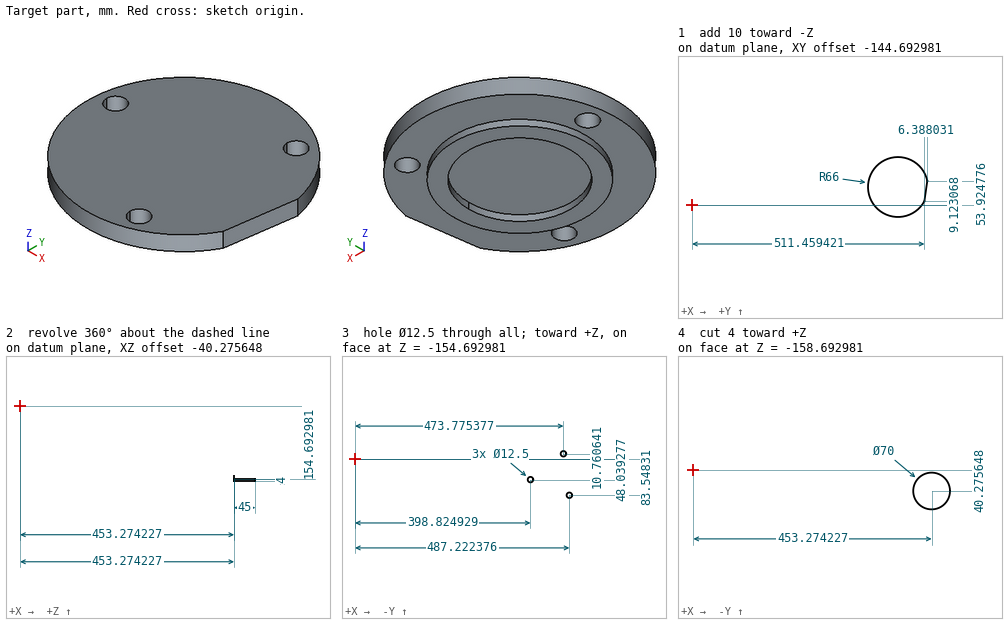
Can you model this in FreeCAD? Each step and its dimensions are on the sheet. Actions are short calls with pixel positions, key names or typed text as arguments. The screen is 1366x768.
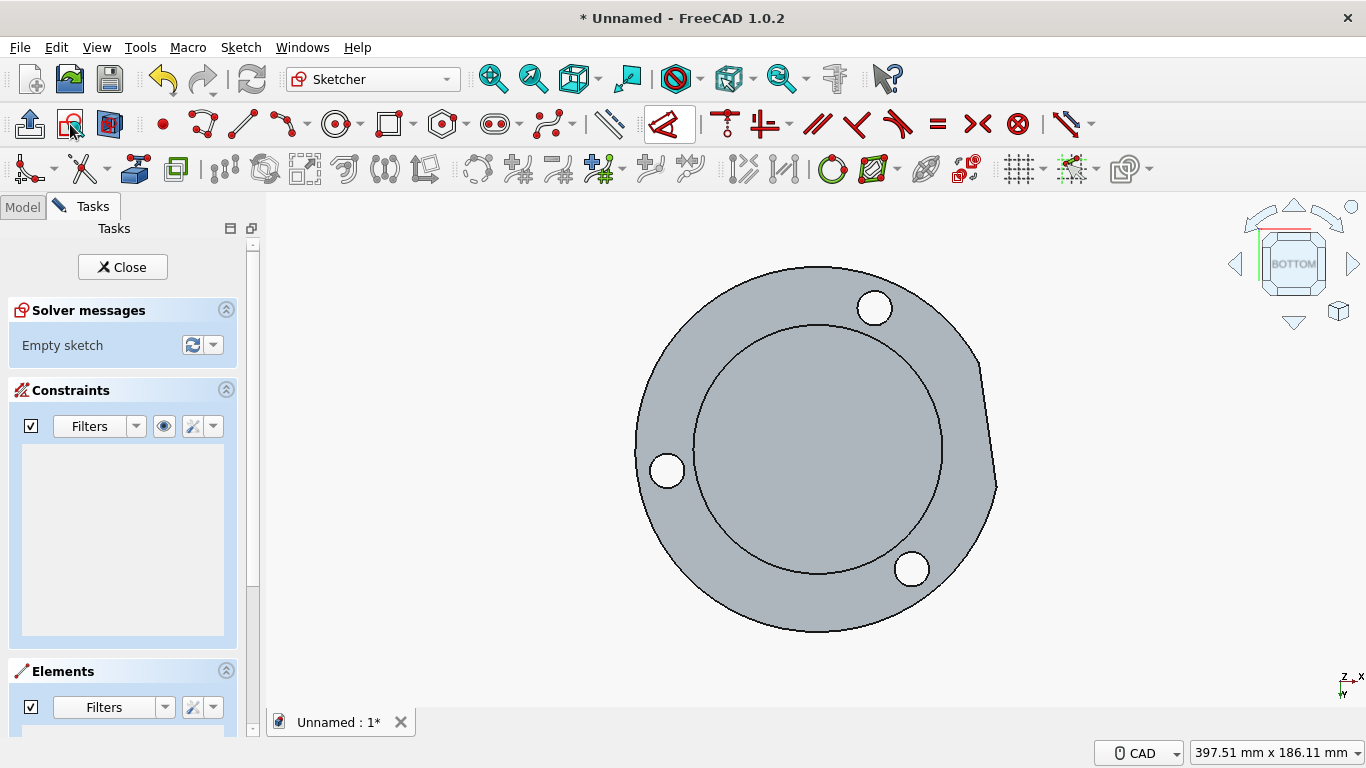
scroll(904, 449, up, 3)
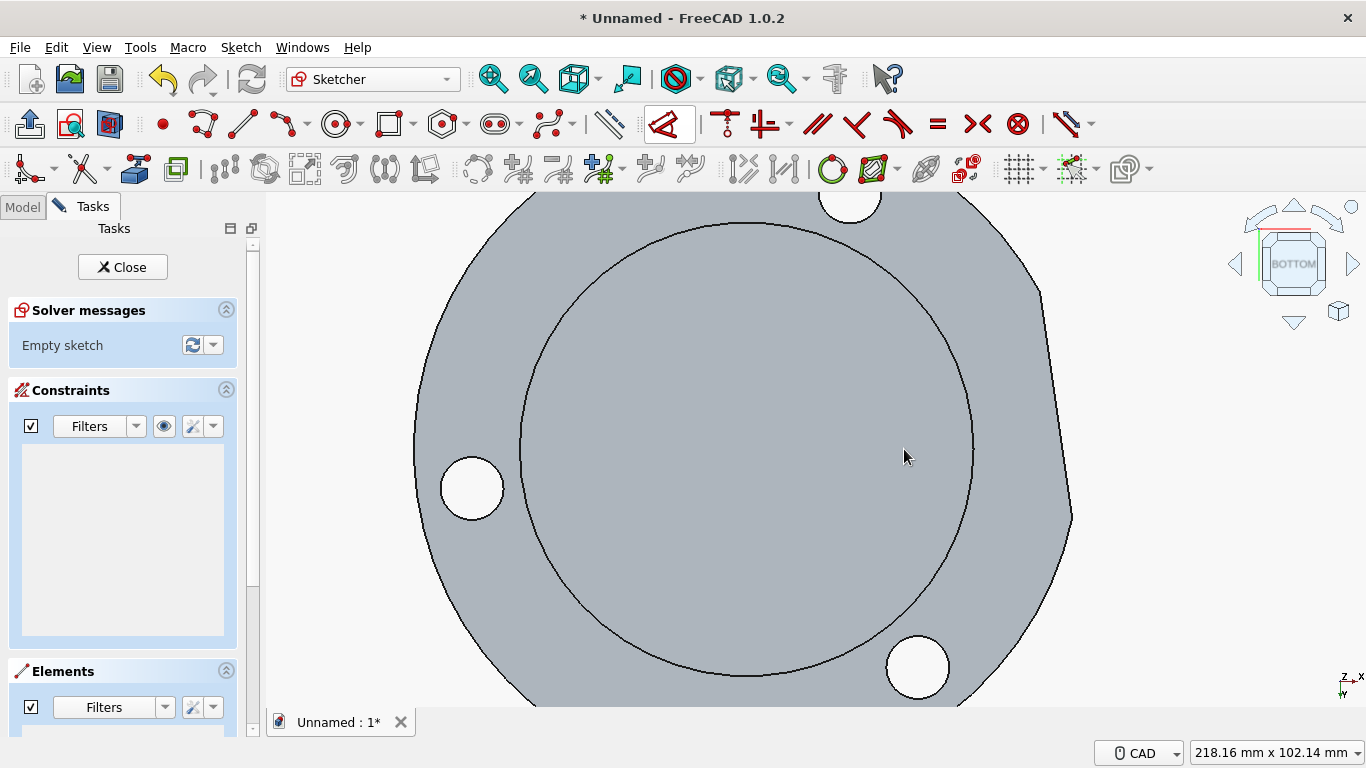
key(g)
key(c)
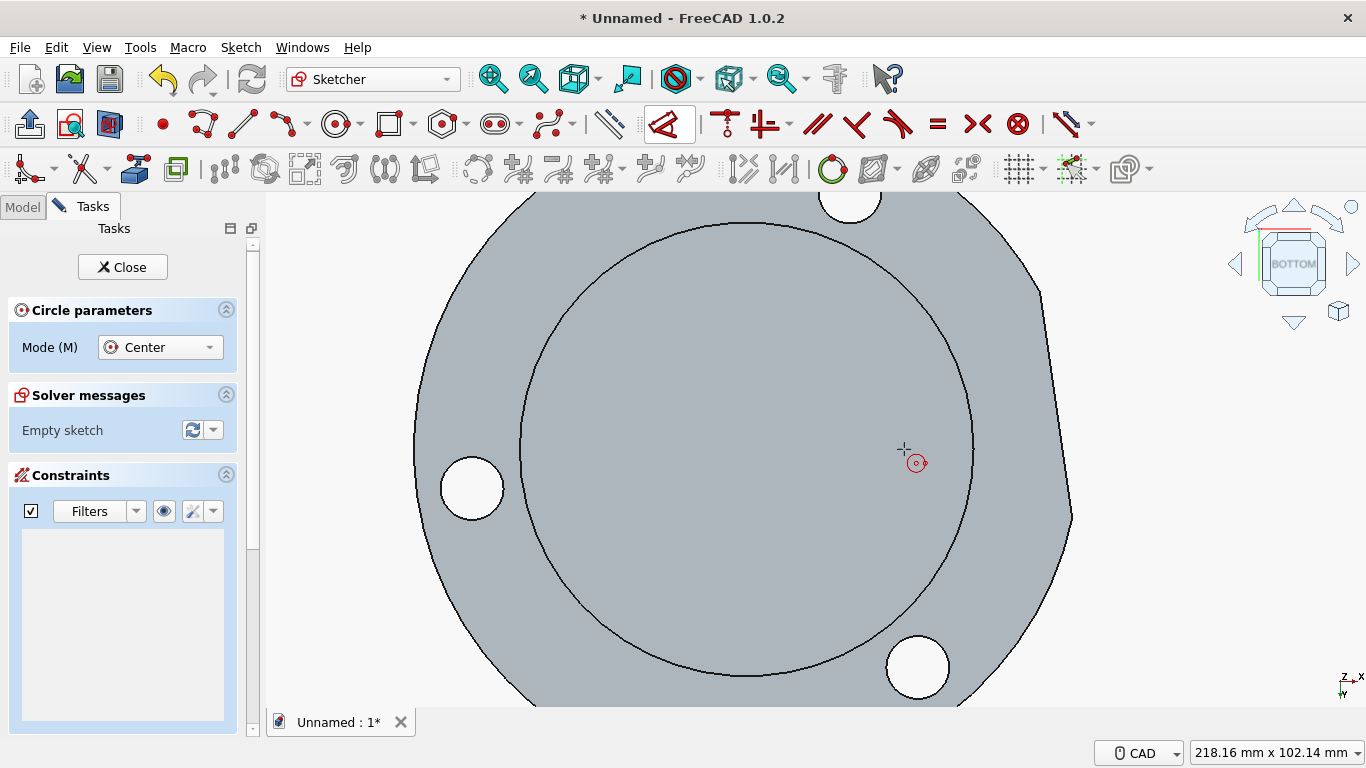
click(747, 449)
move(871, 325)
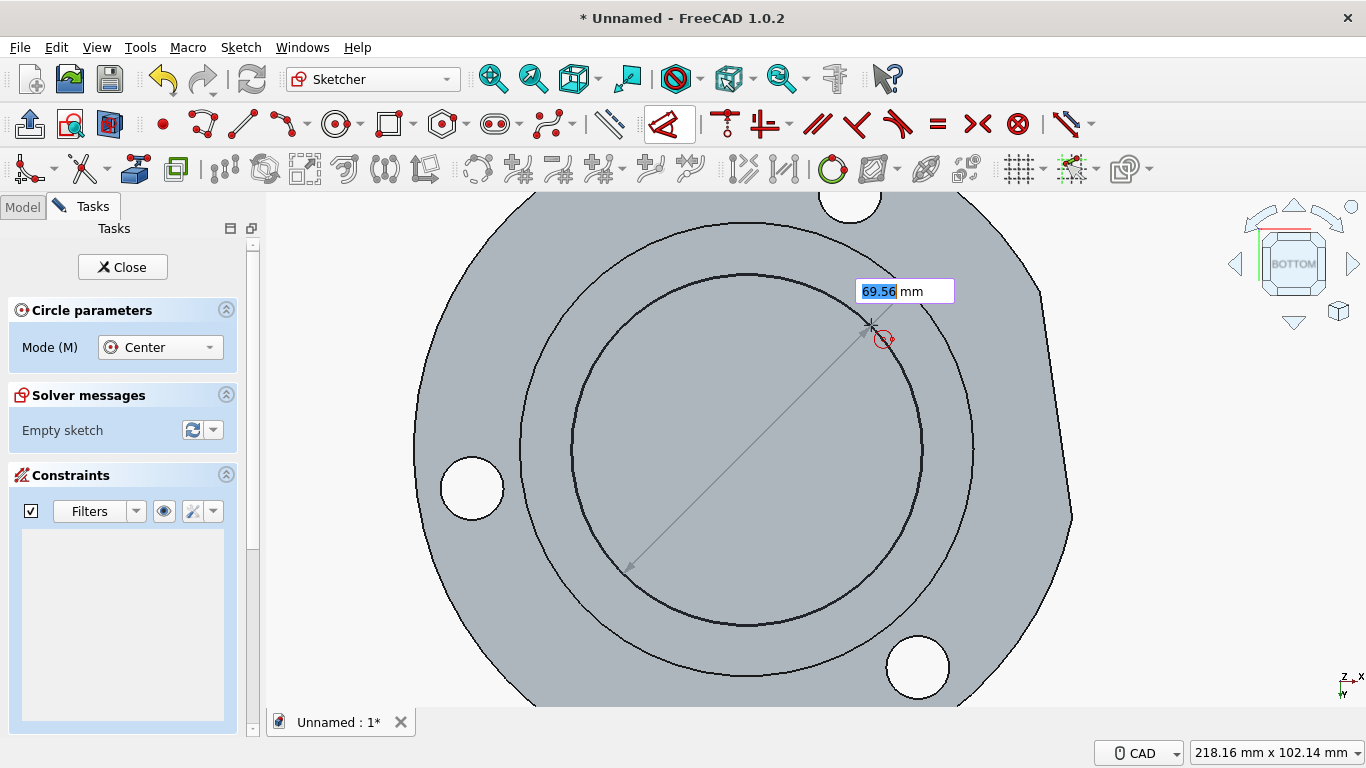
text(70)
key(Return)
key(Escape)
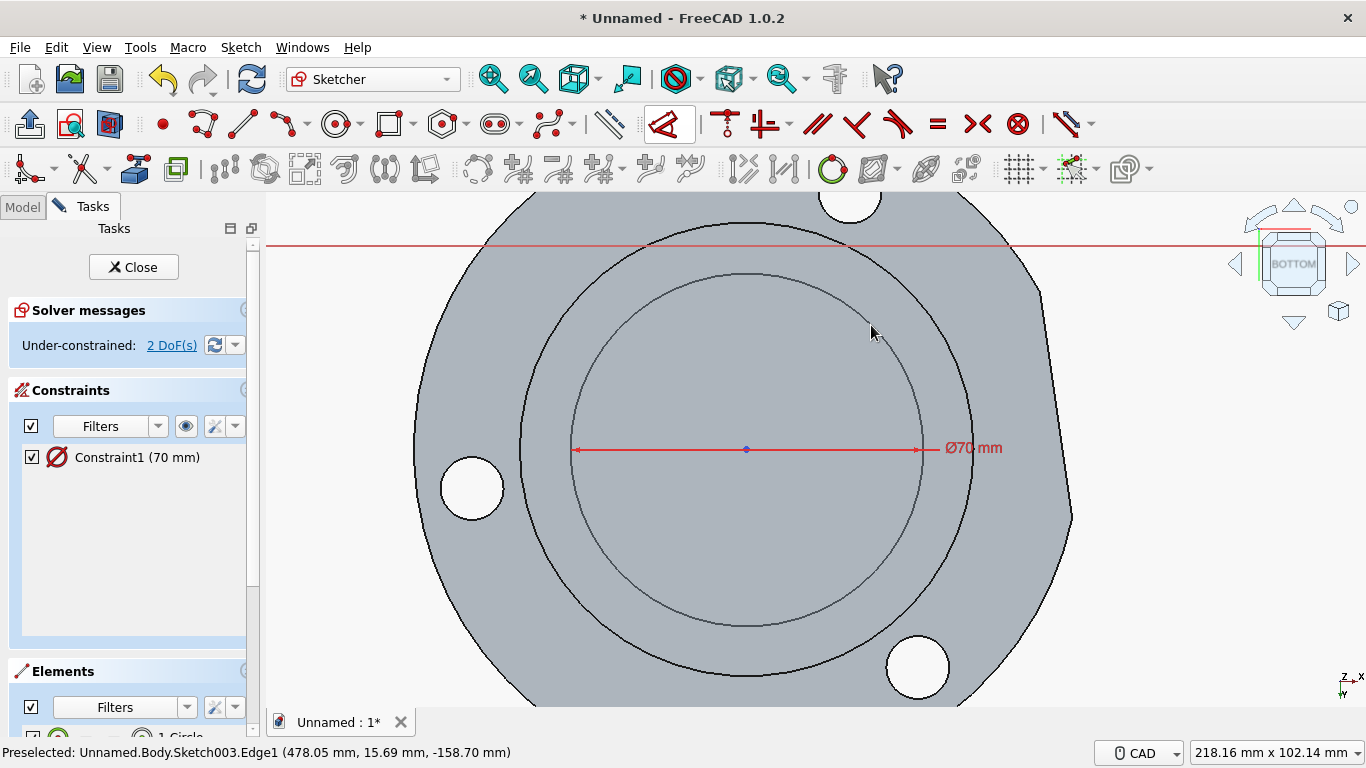
click(747, 450)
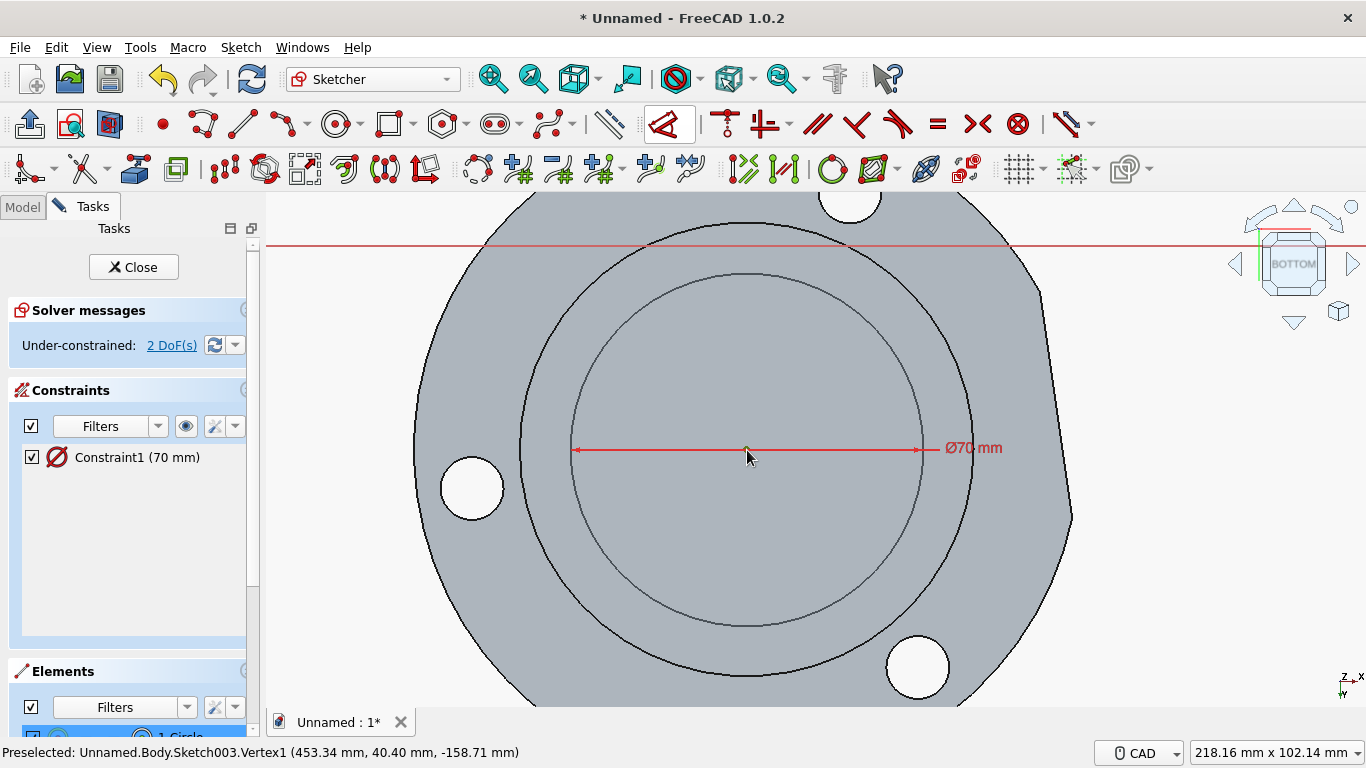
key(i)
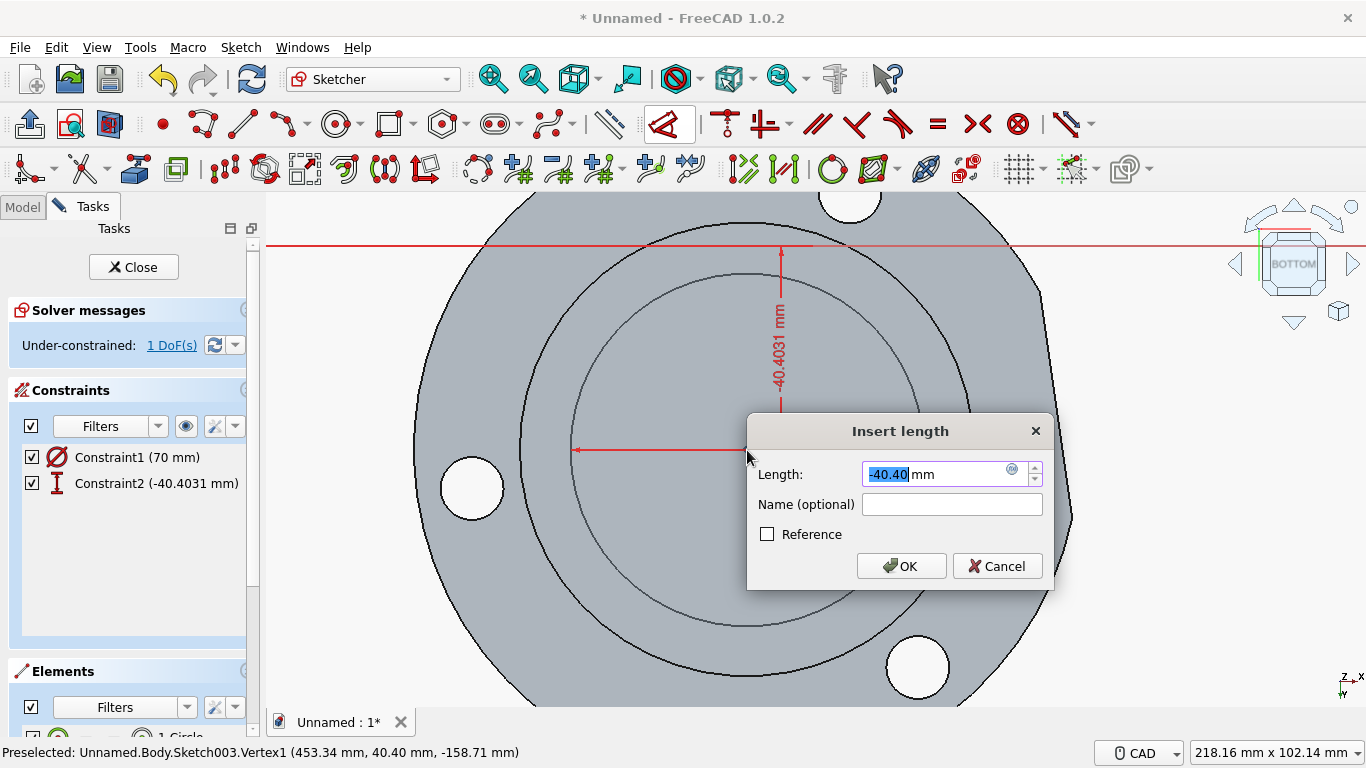
text(-40.275648)
key(Return)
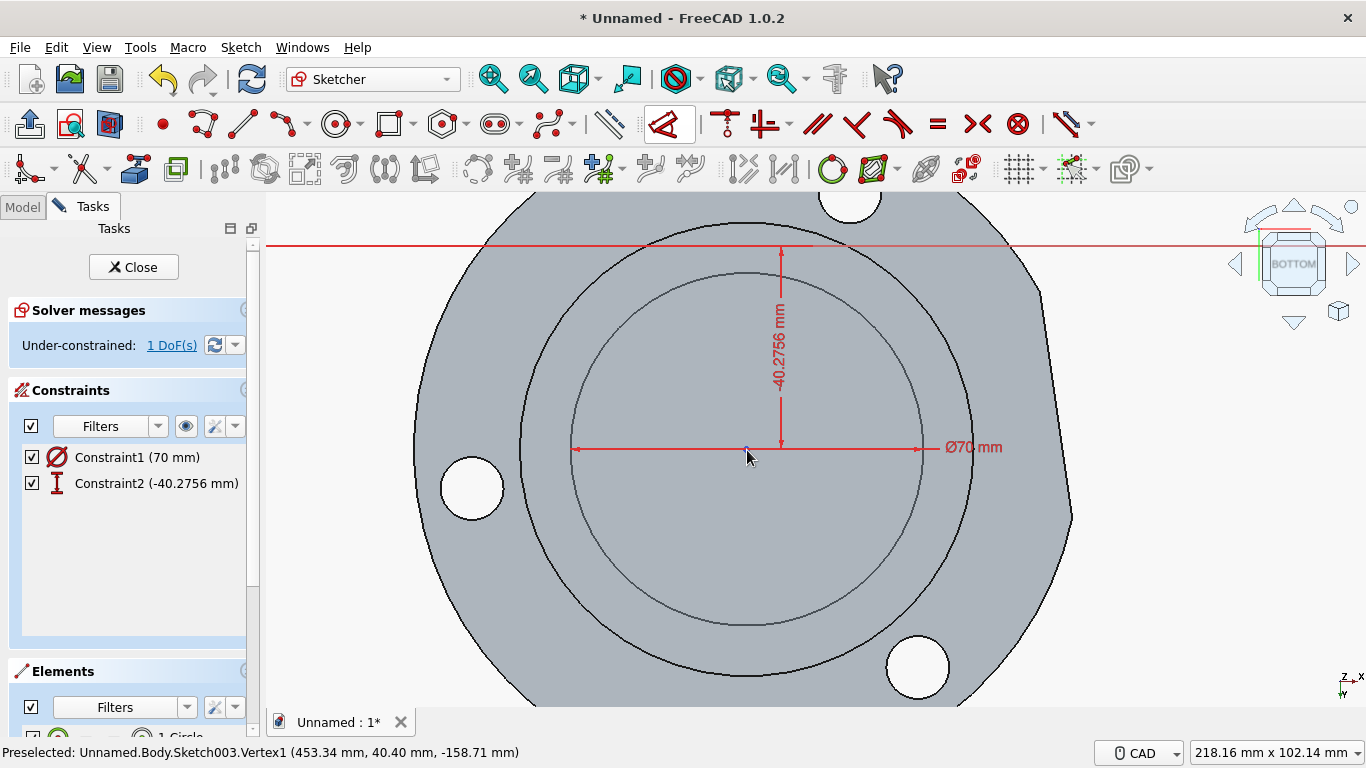
click(747, 449)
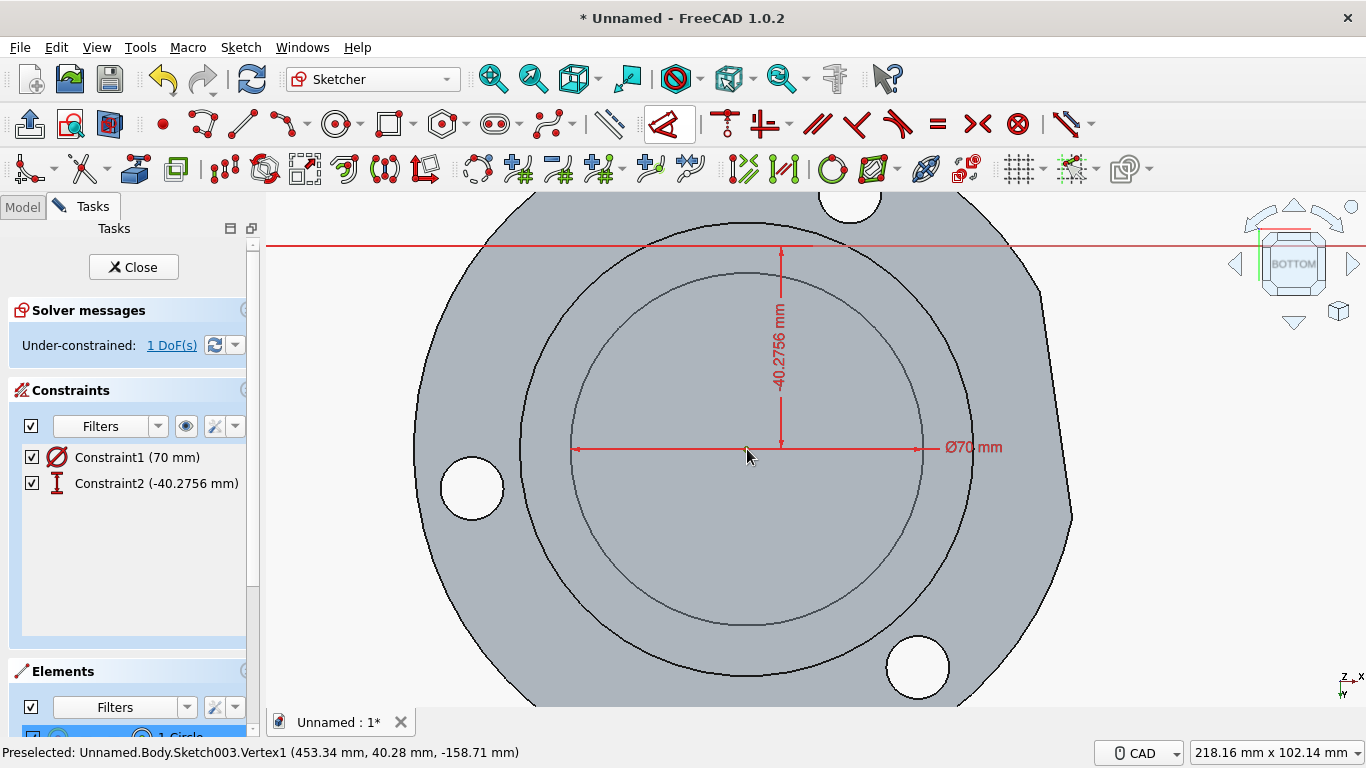
click(690, 124)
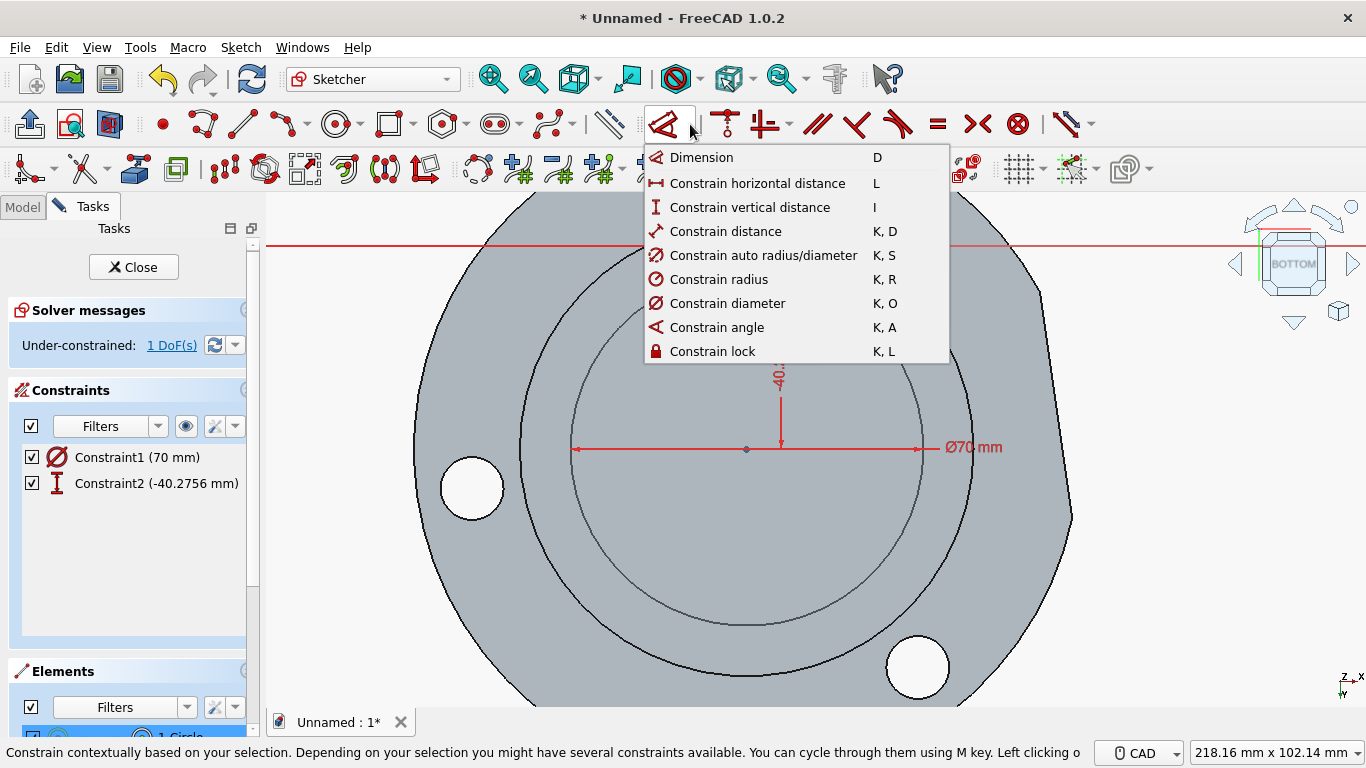
click(797, 183)